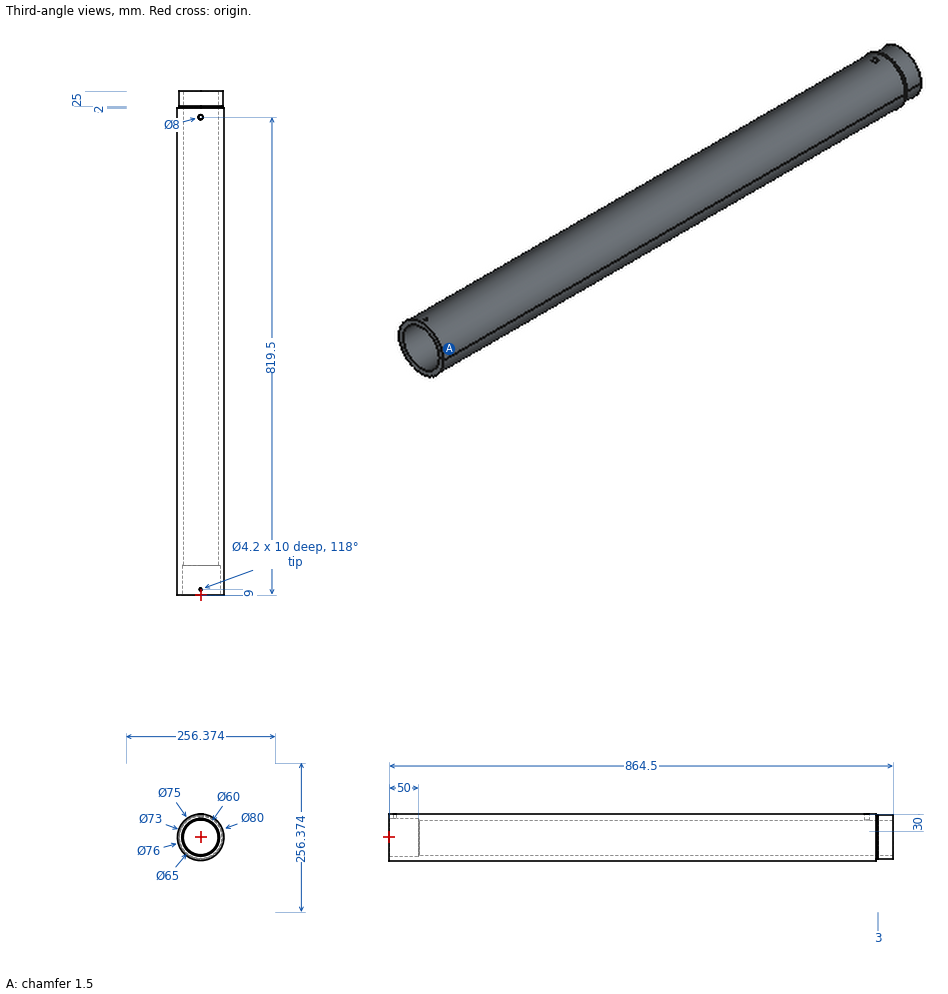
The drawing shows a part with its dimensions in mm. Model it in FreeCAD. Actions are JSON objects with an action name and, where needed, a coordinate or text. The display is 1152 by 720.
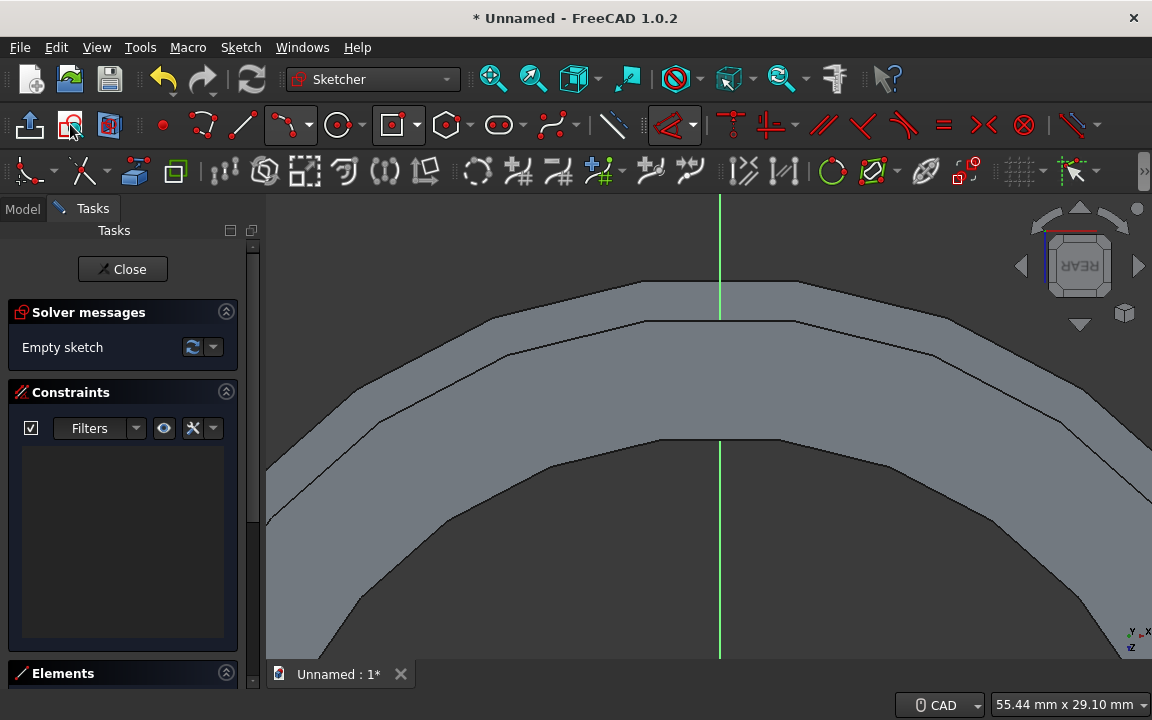
{"action": "left_click", "coordinate": [110, 126]}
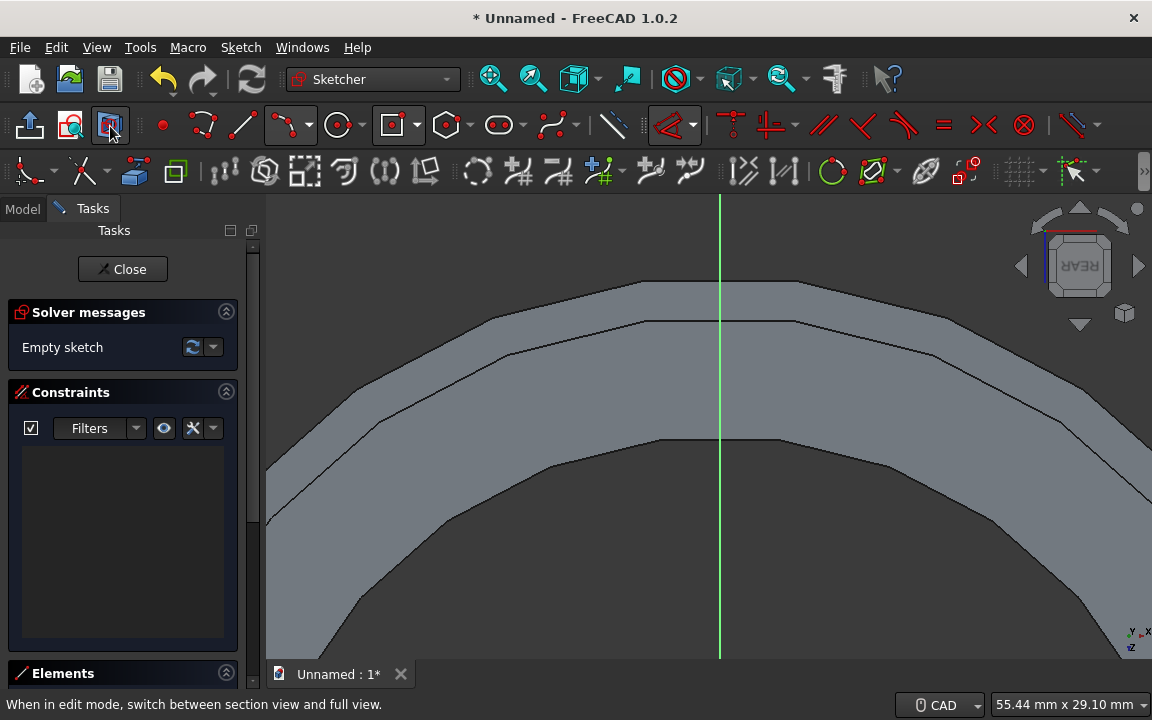
{"action": "scroll", "coordinate": [634, 387], "scroll_direction": "down", "scroll_amount": 13}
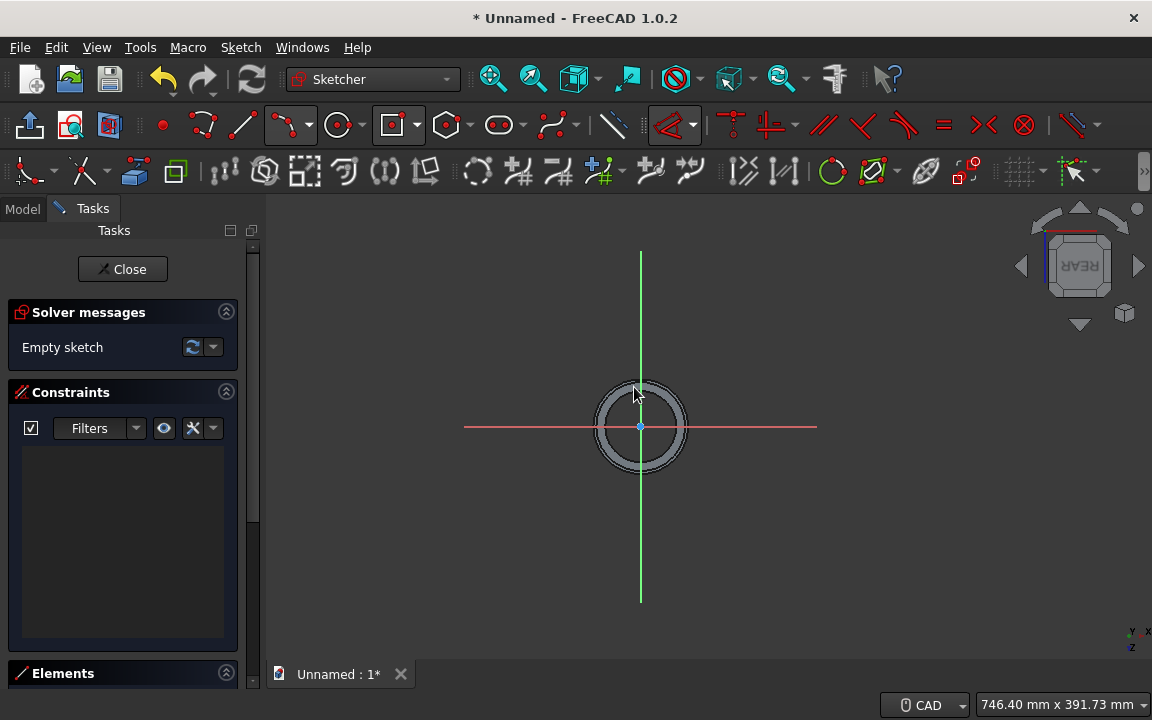
{"action": "left_click", "coordinate": [392, 126]}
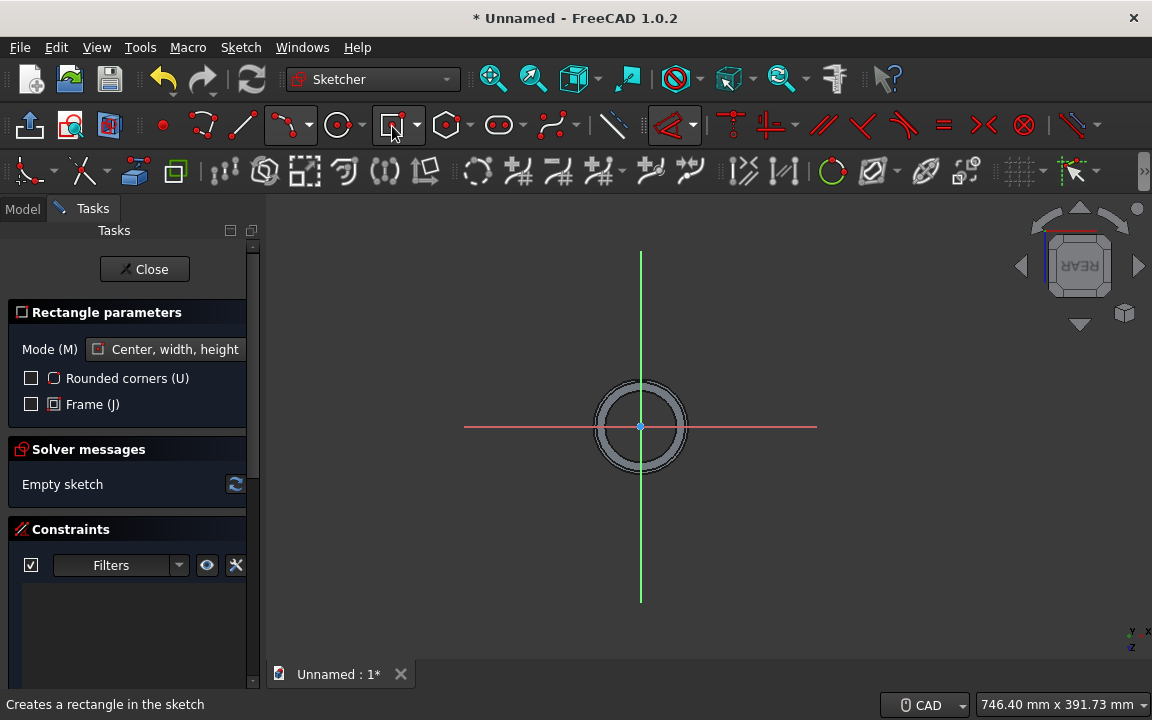
{"action": "left_click", "coordinate": [641, 427]}
{"action": "mouse_move", "coordinate": [793, 274]}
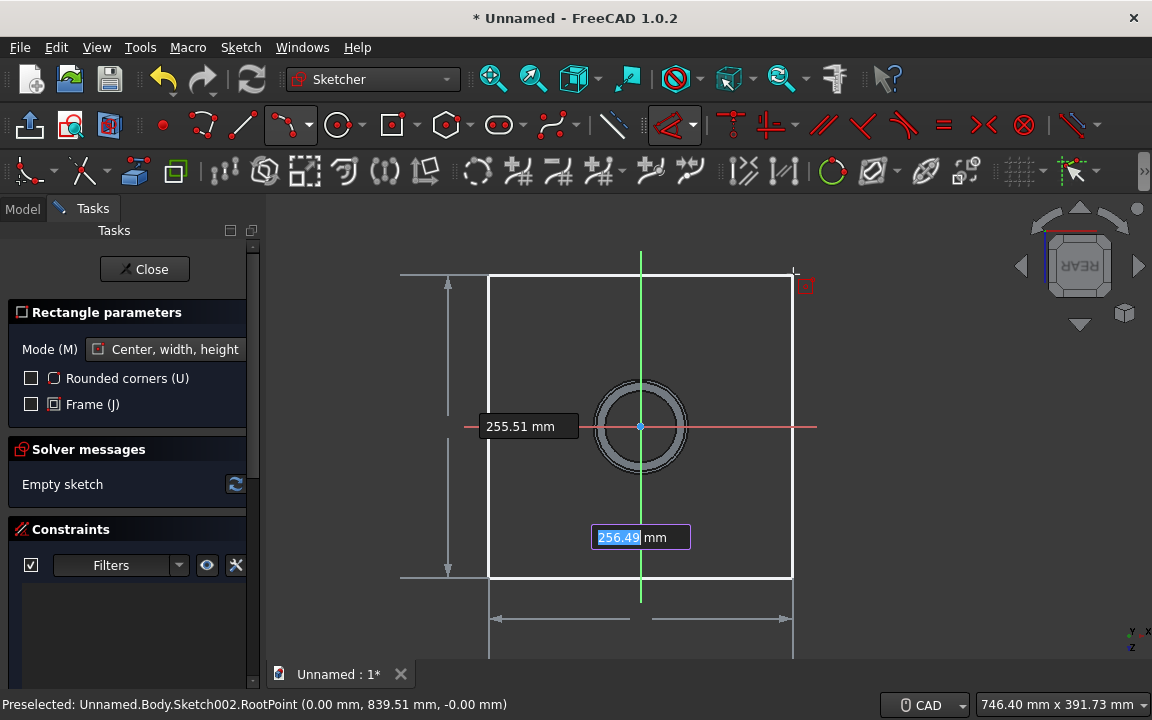
{"action": "type", "text": "256.374"}
{"action": "key", "text": "Tab"}
{"action": "type", "text": "256.374"}
{"action": "key", "text": "Return"}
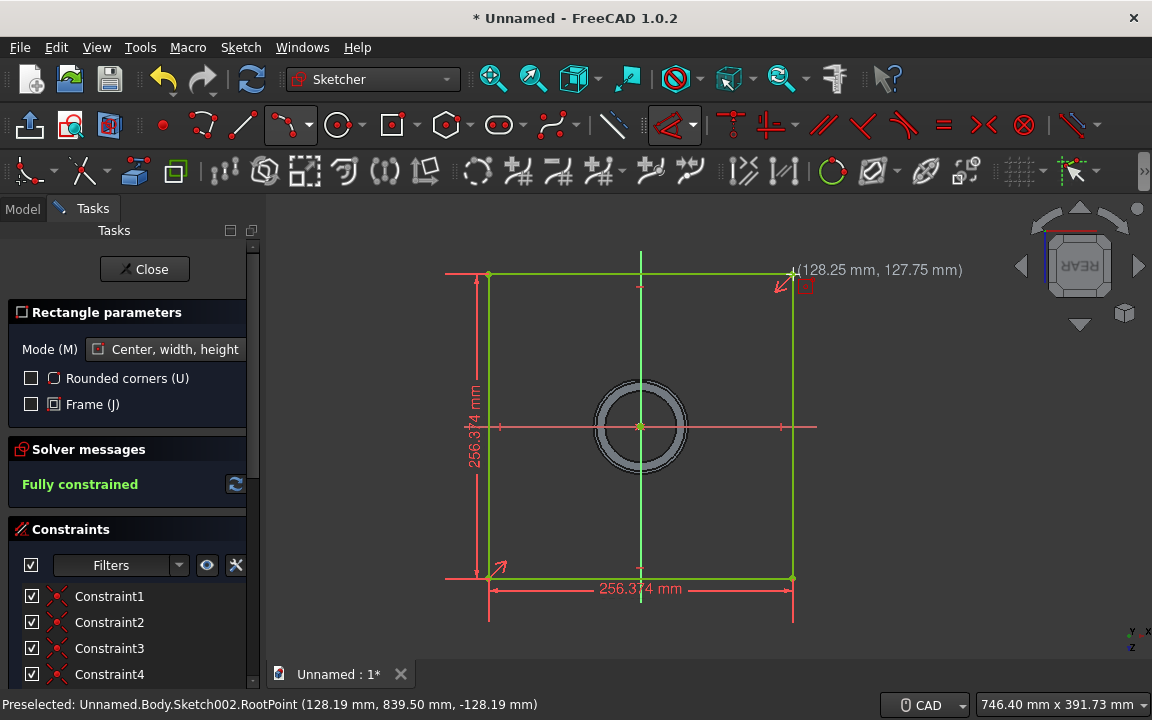
{"action": "left_click", "coordinate": [338, 126]}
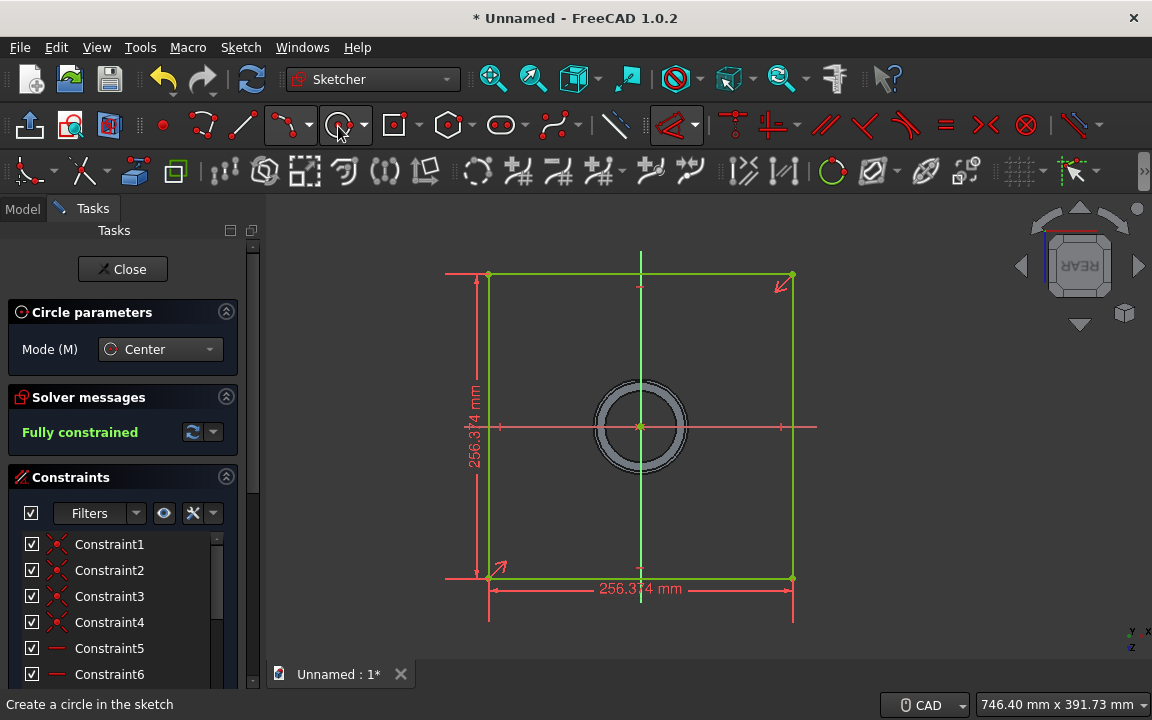
{"action": "left_click", "coordinate": [641, 427]}
{"action": "mouse_move", "coordinate": [671, 396]}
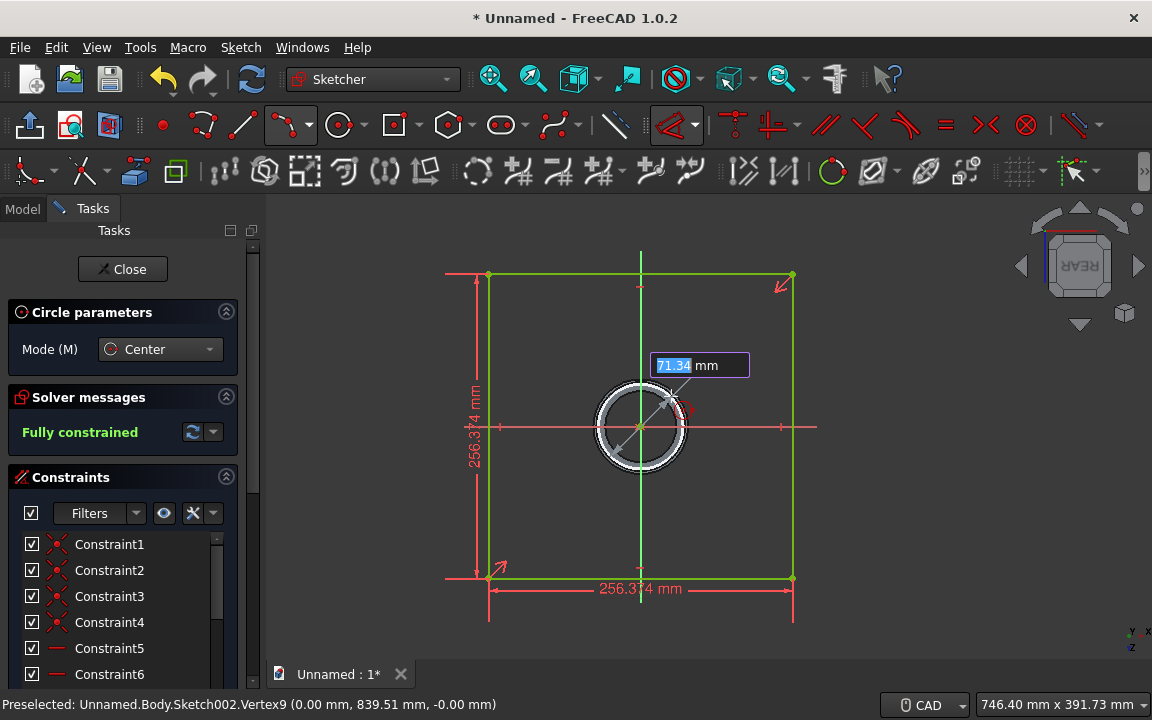
{"action": "type", "text": "73"}
{"action": "key", "text": "Return"}
{"action": "key", "text": "Escape"}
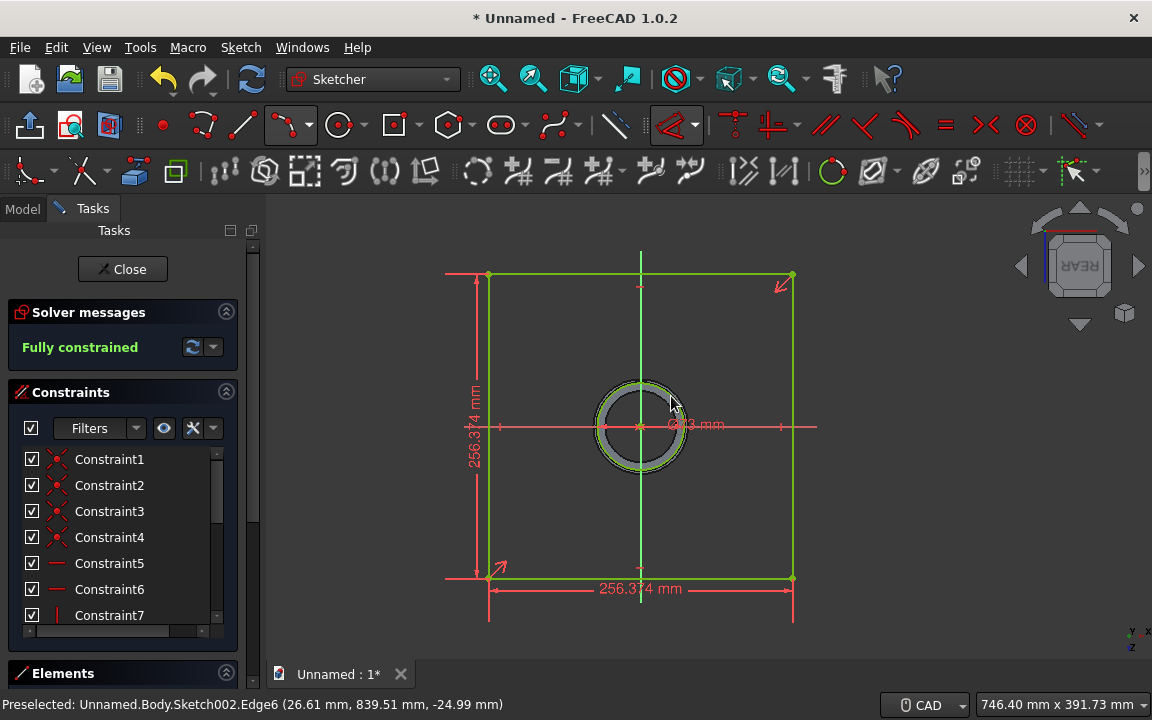
{"action": "left_click", "coordinate": [123, 269]}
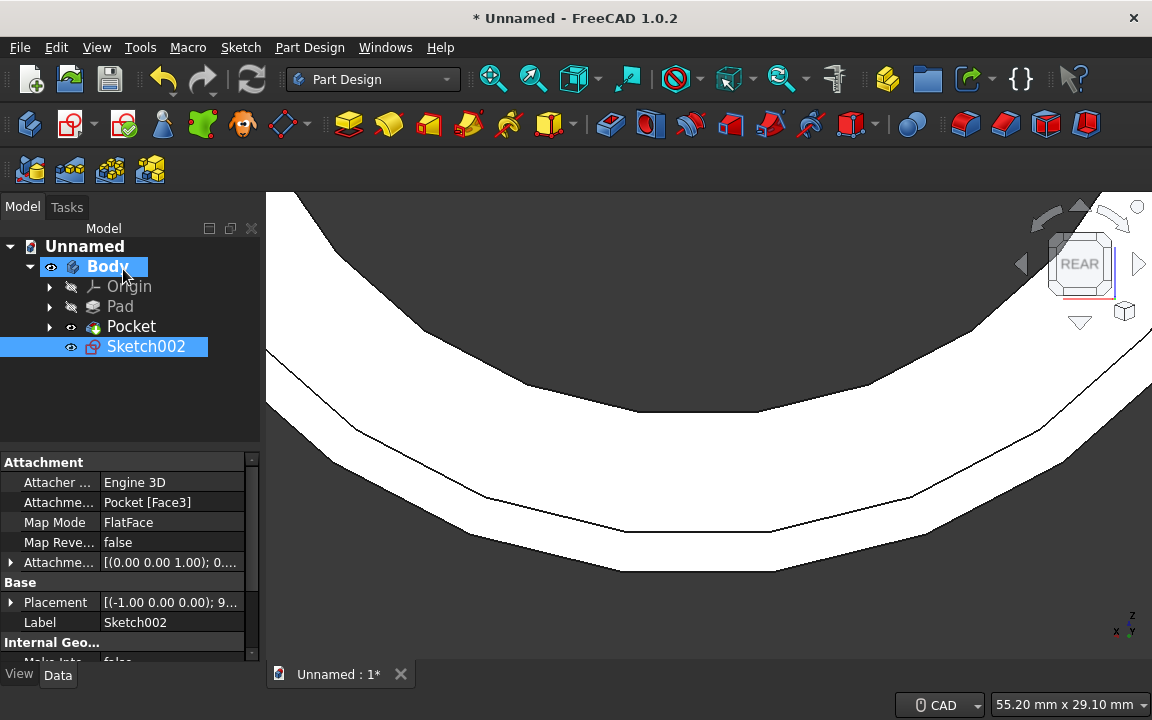
{"action": "left_click", "coordinate": [612, 124]}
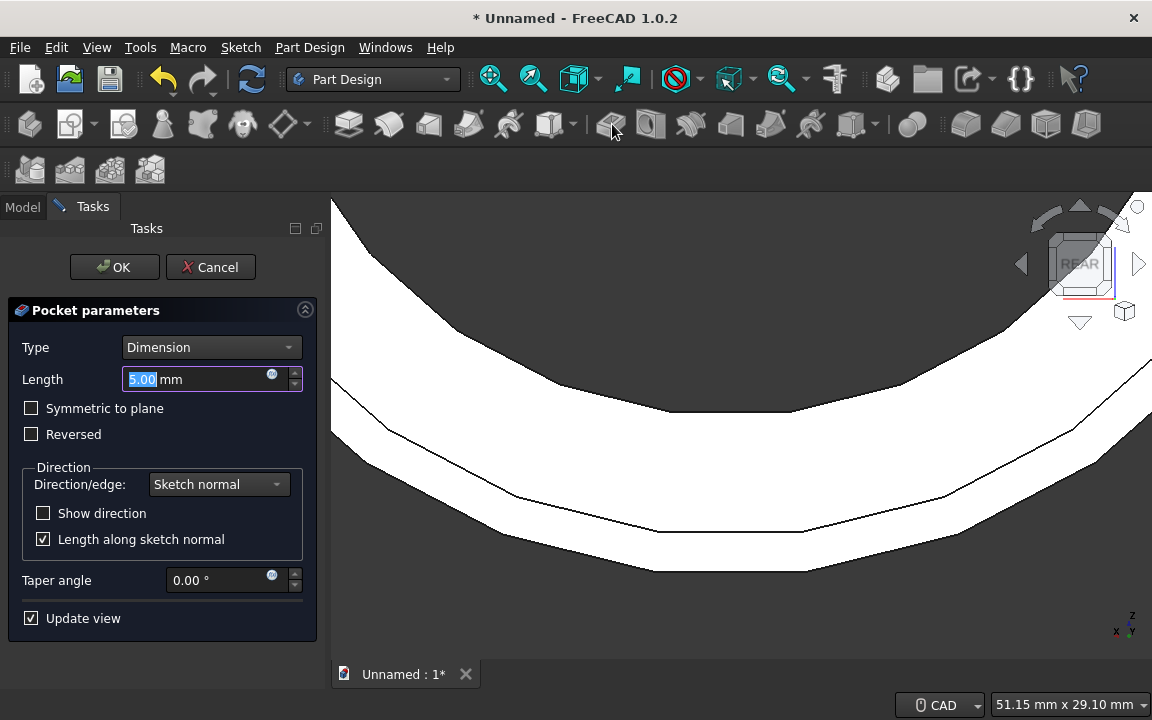
{"action": "type", "text": "3"}
{"action": "key", "text": "Tab"}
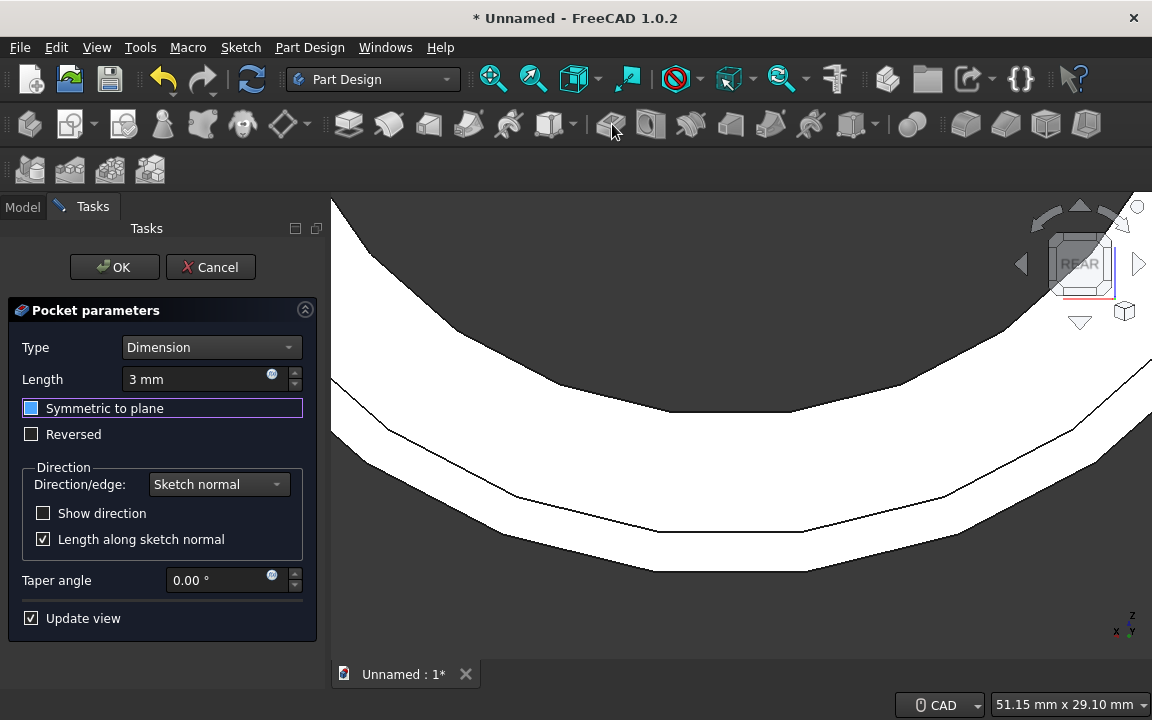
{"action": "left_click", "coordinate": [115, 267]}